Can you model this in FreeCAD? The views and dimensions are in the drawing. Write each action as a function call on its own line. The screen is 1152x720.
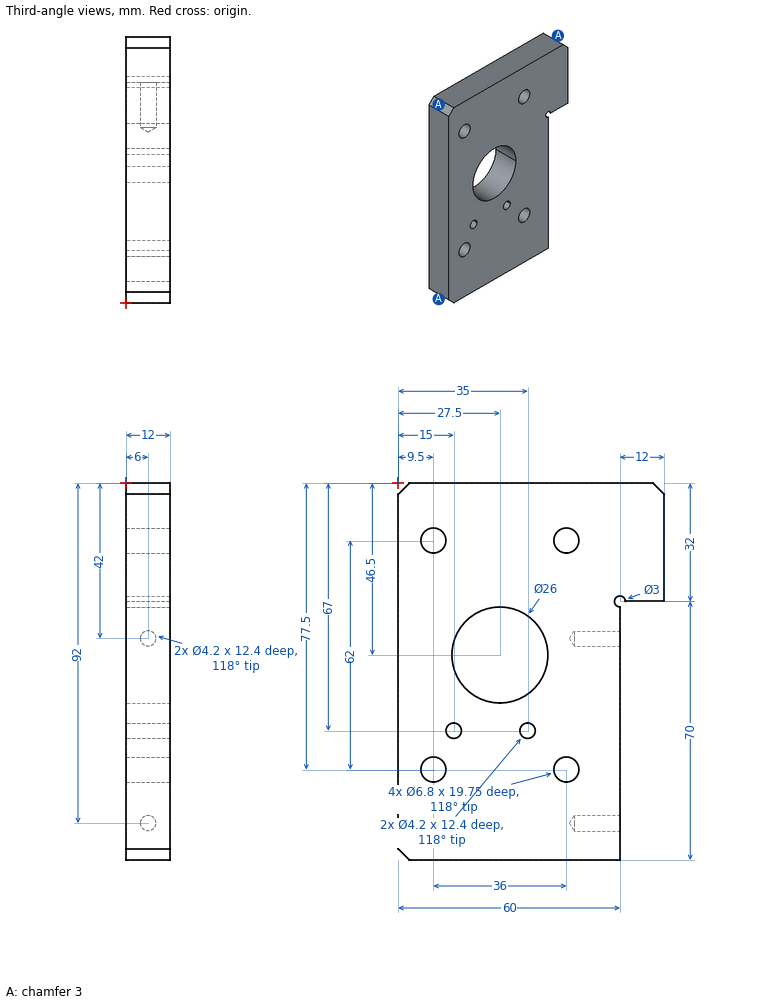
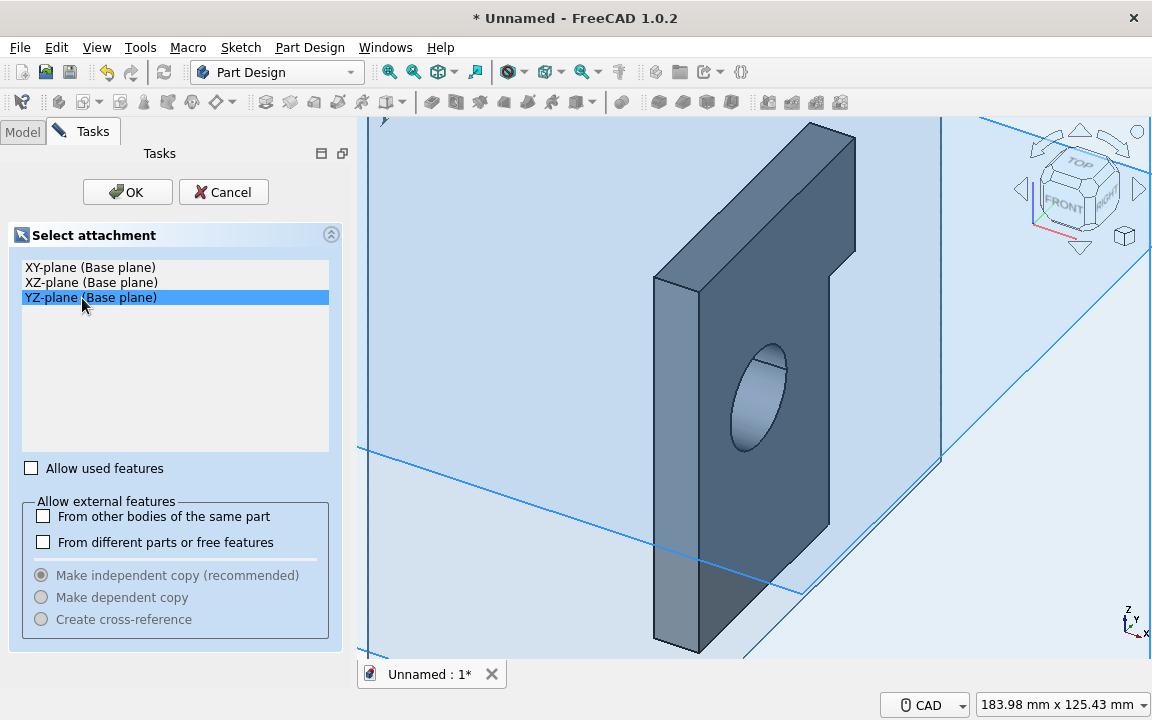
click(128, 192)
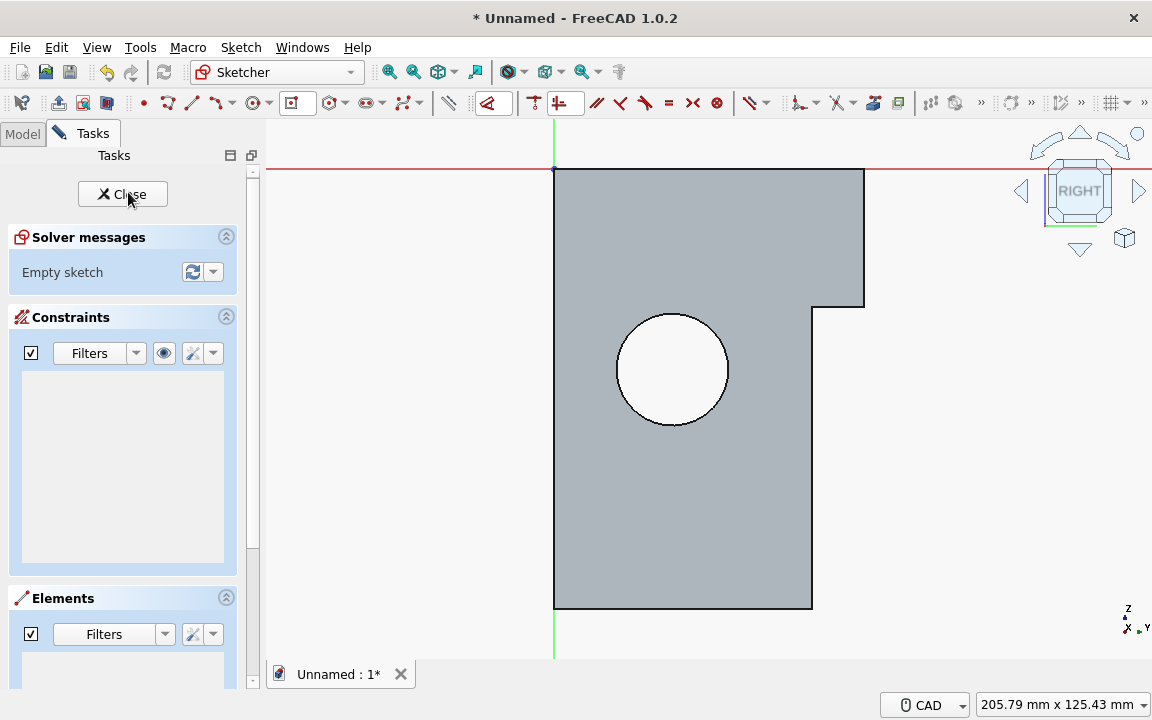
click(108, 104)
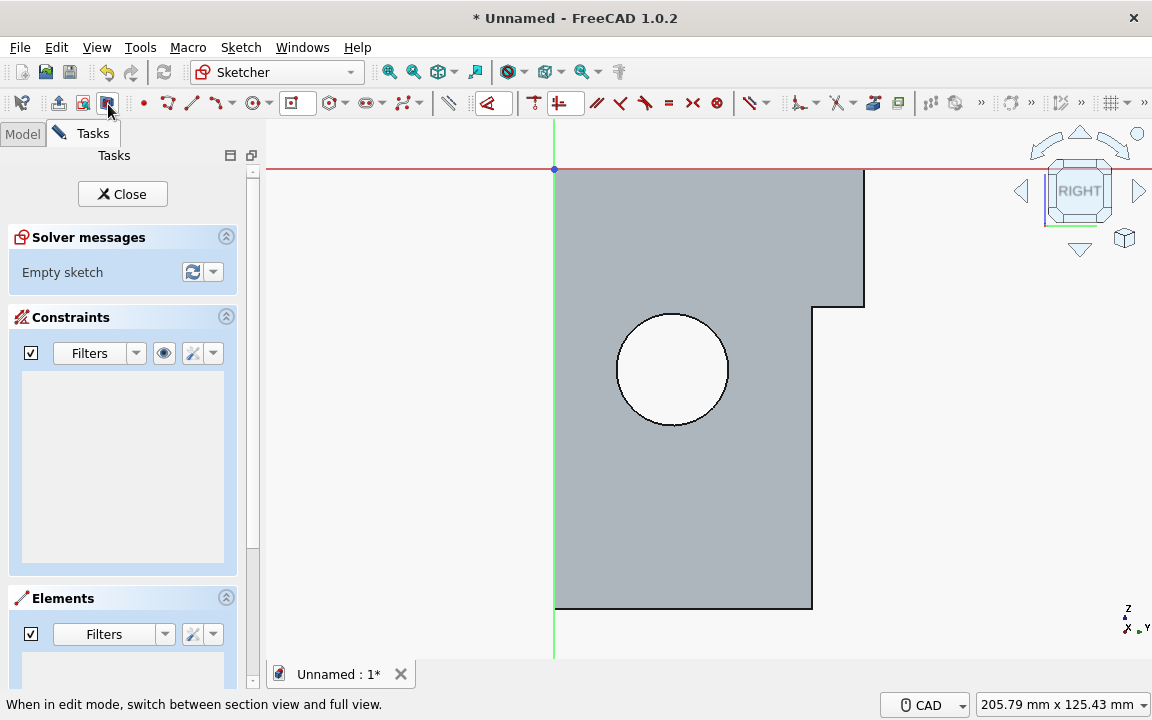
scroll(556, 594, down, 1)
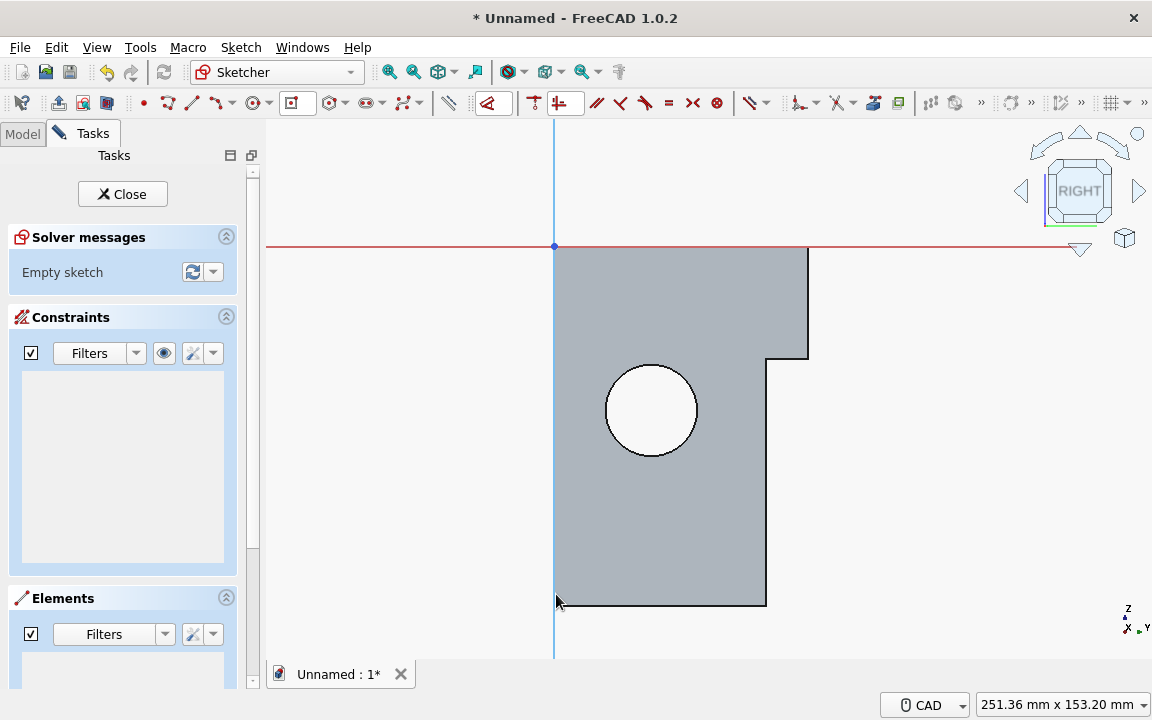
click(254, 104)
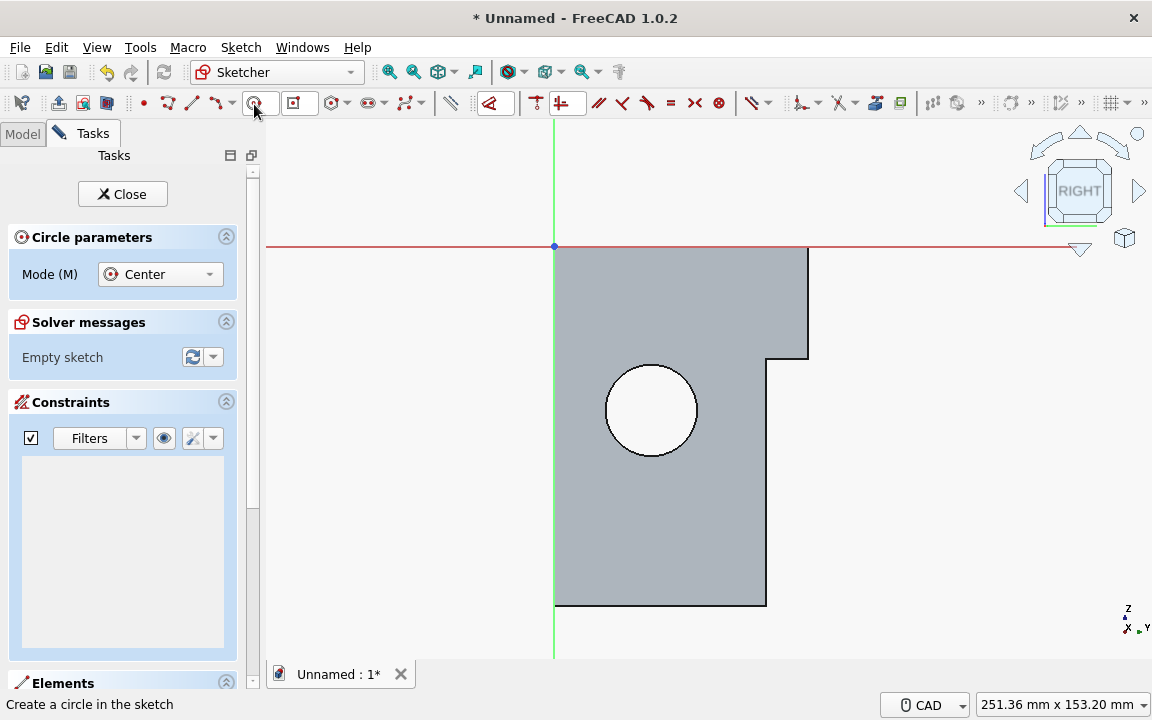
scroll(715, 520, up, 4)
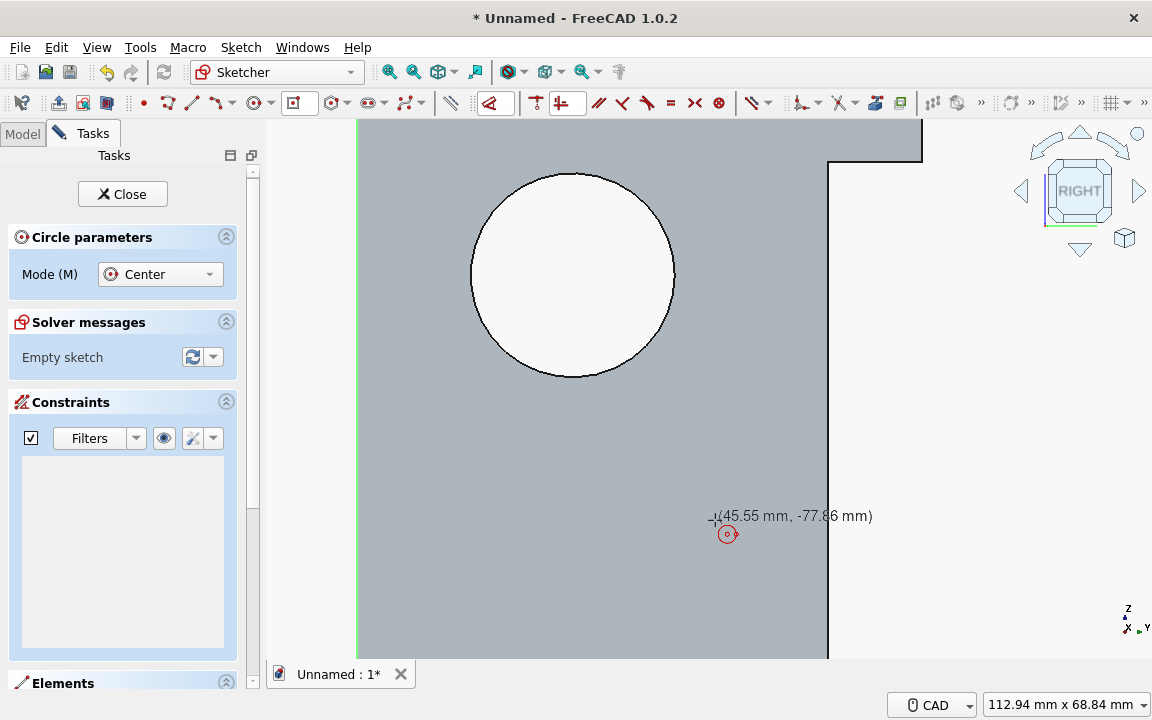
click(714, 518)
move(733, 500)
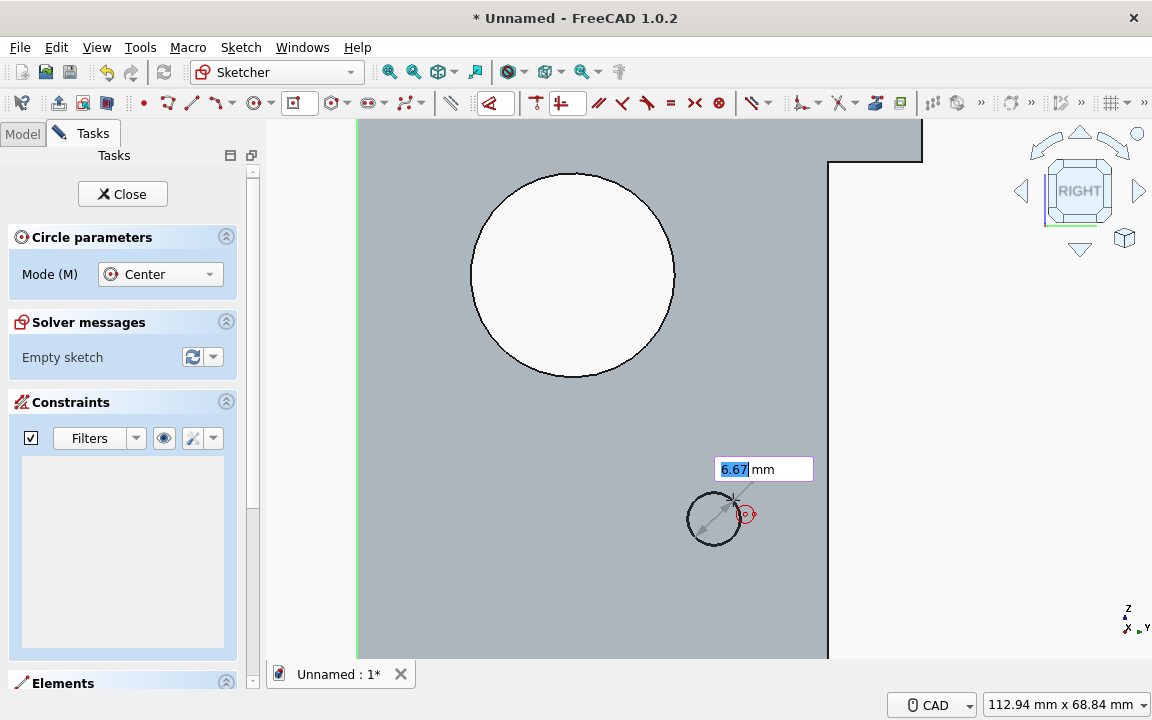
text(6.8)
key(Return)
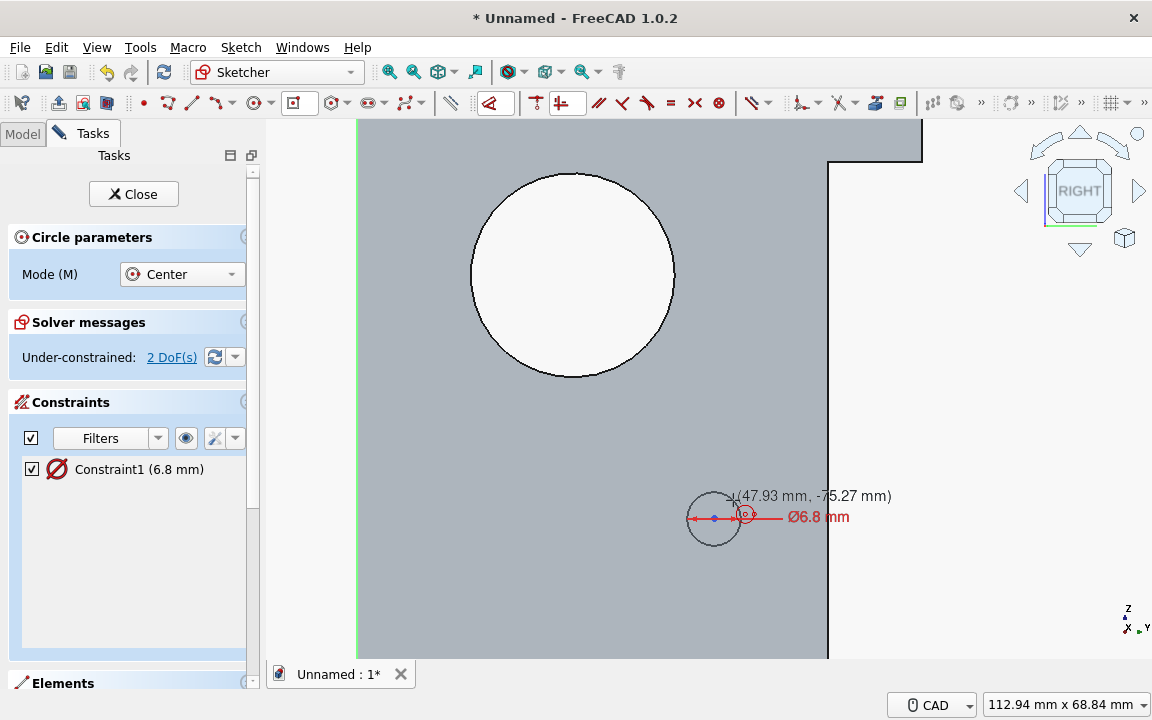
click(432, 518)
move(450, 500)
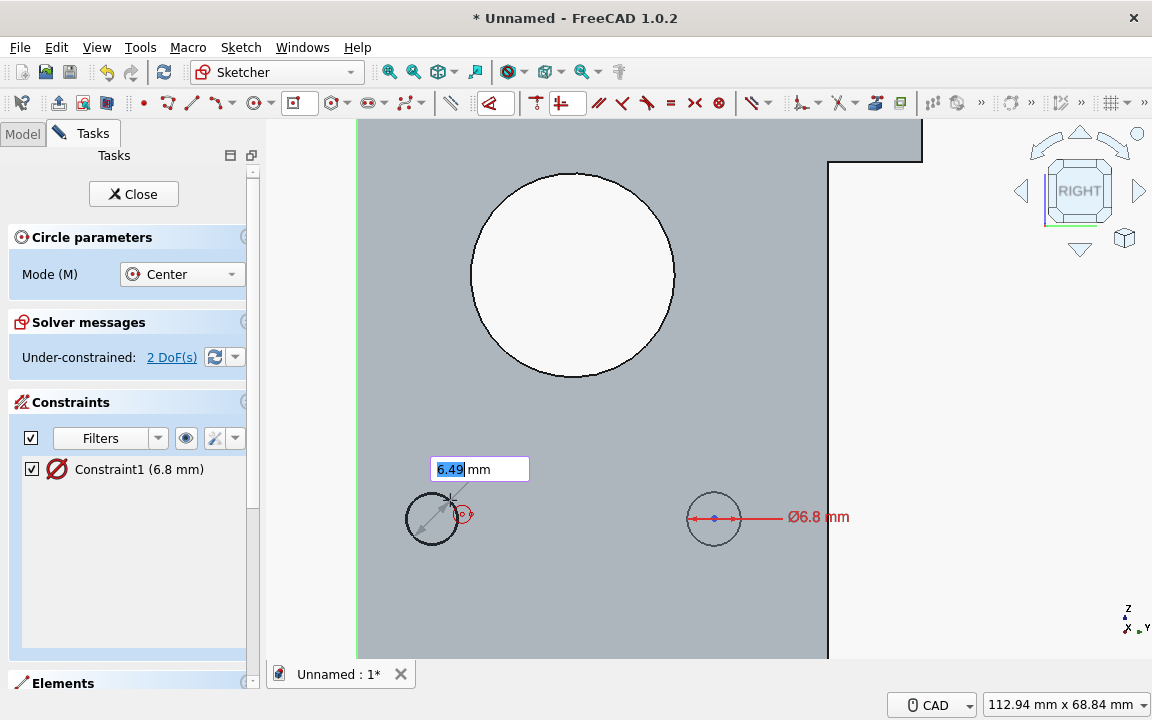
text(6.8)
key(Return)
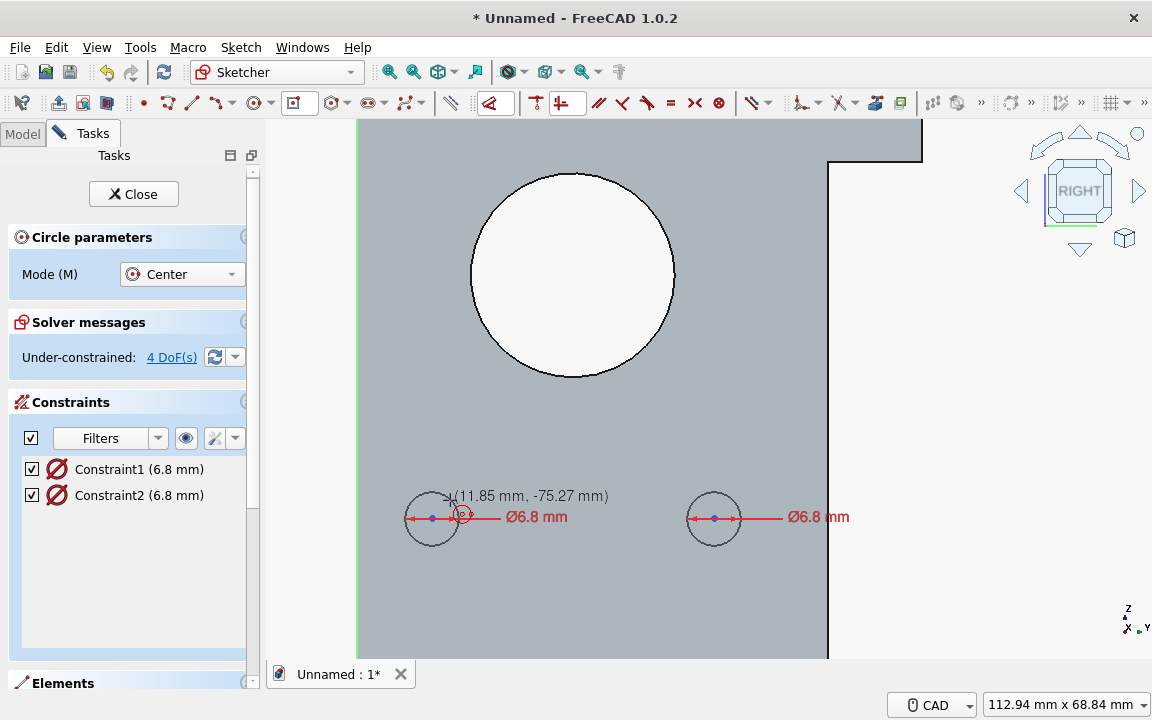
scroll(752, 585, down, 3)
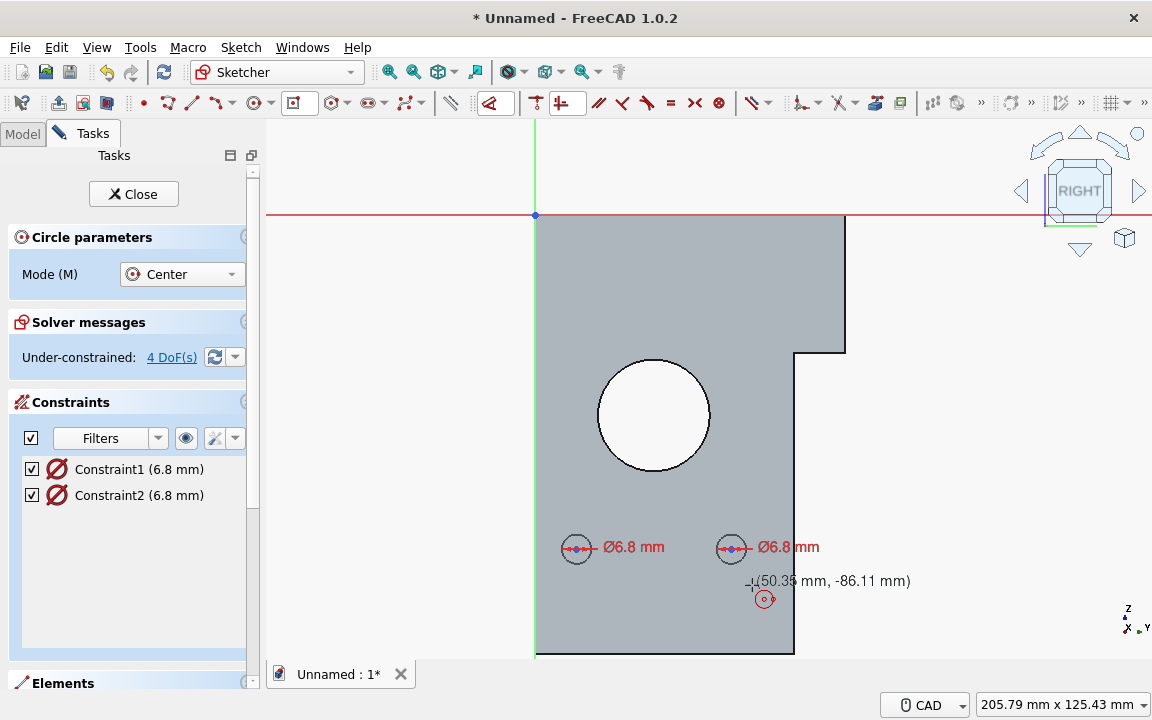
scroll(576, 282, up, 3)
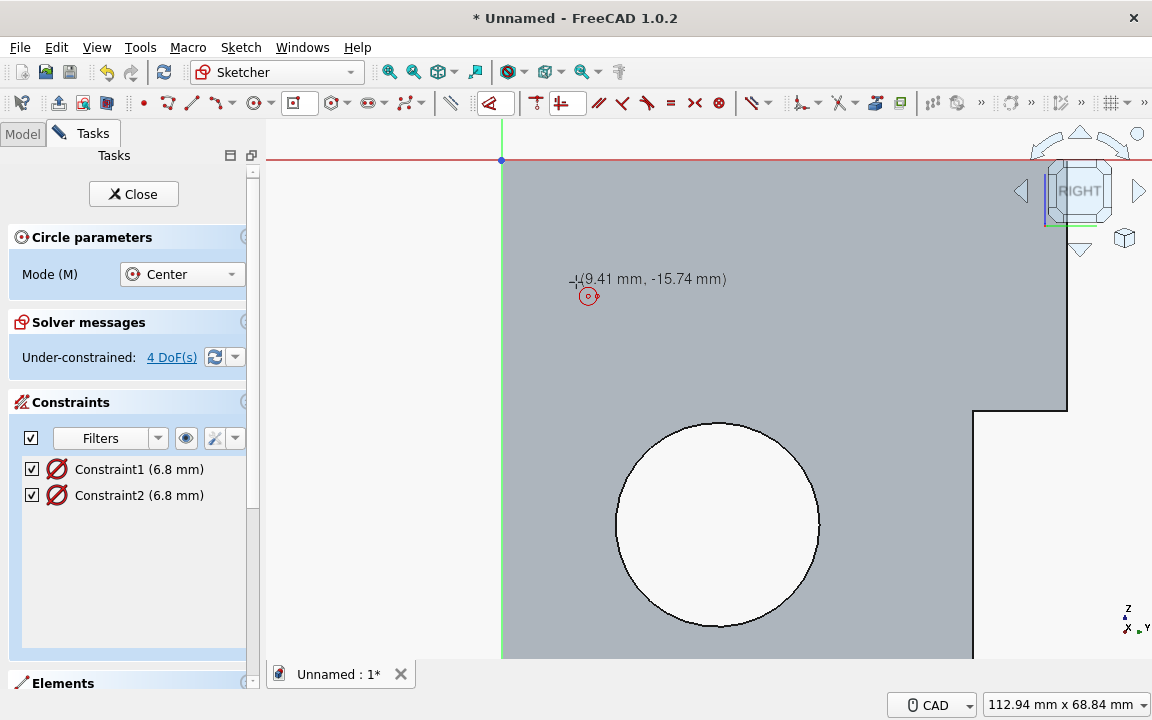
click(576, 282)
move(595, 263)